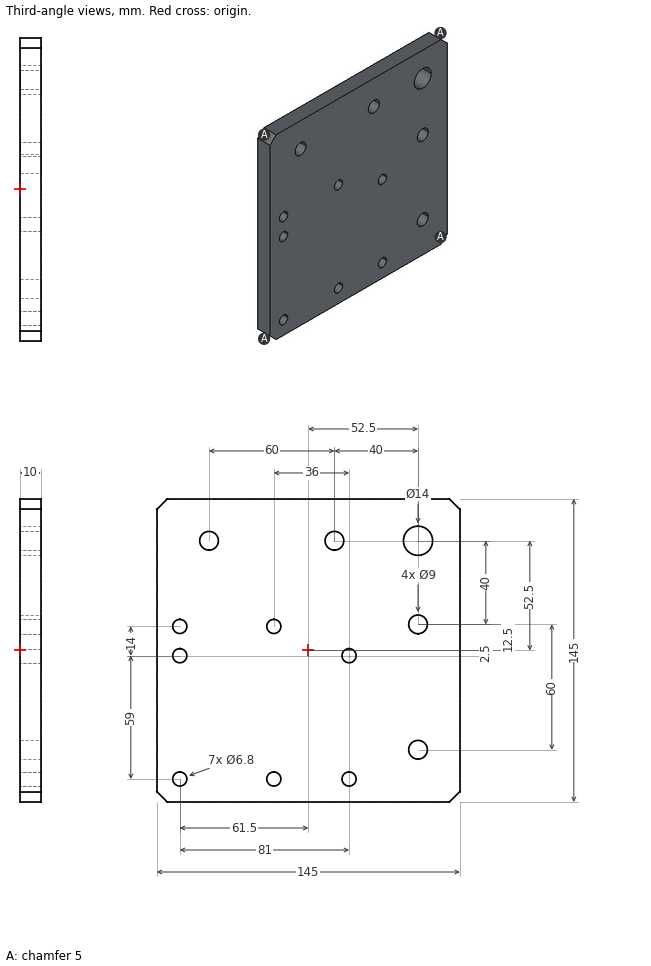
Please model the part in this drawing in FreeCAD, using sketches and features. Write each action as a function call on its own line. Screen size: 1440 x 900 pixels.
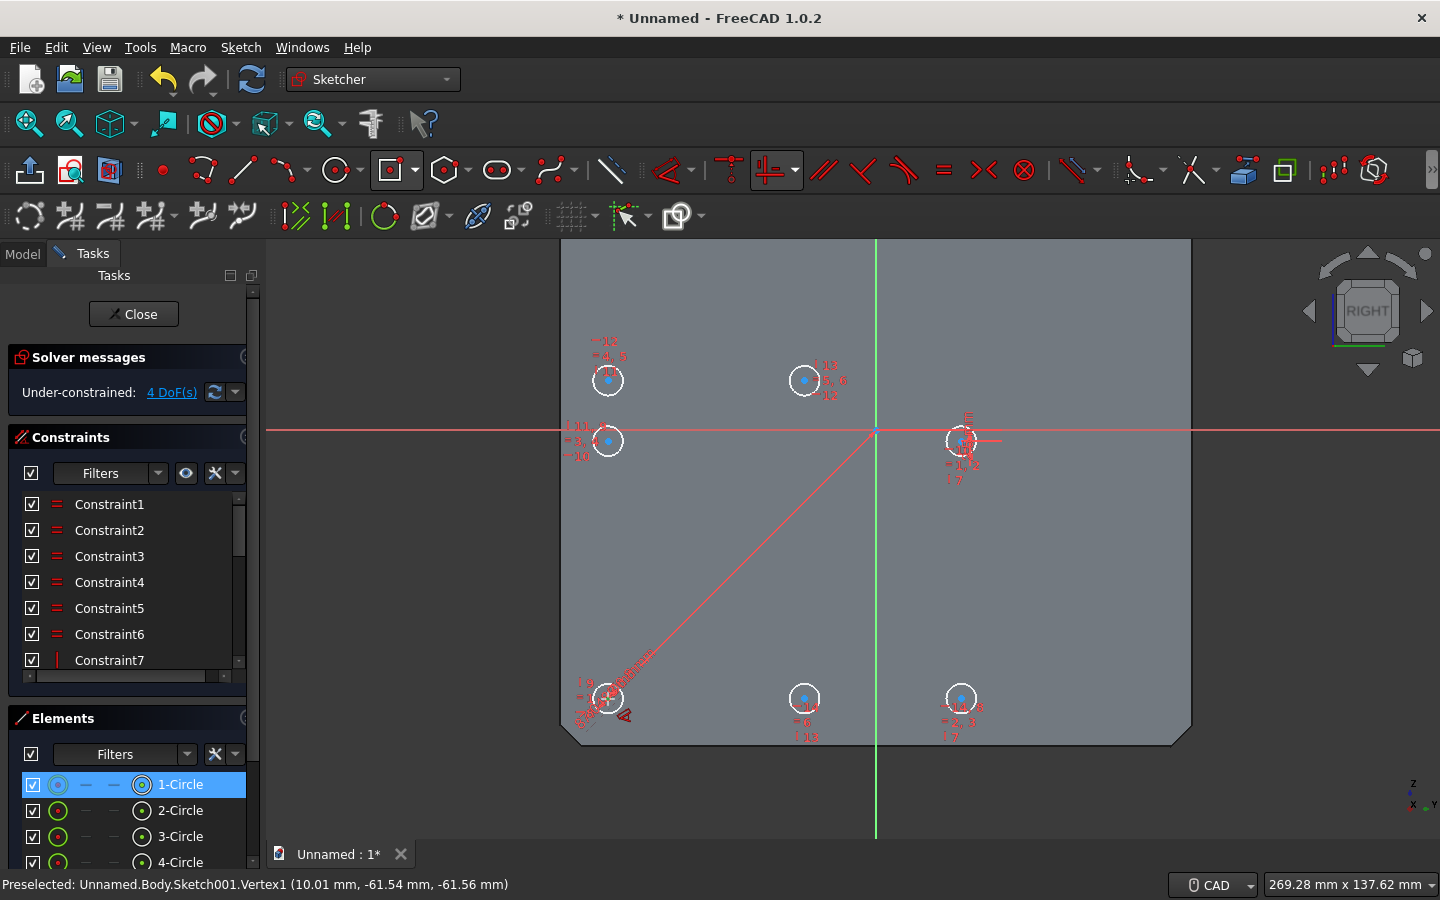
click(961, 441)
click(785, 733)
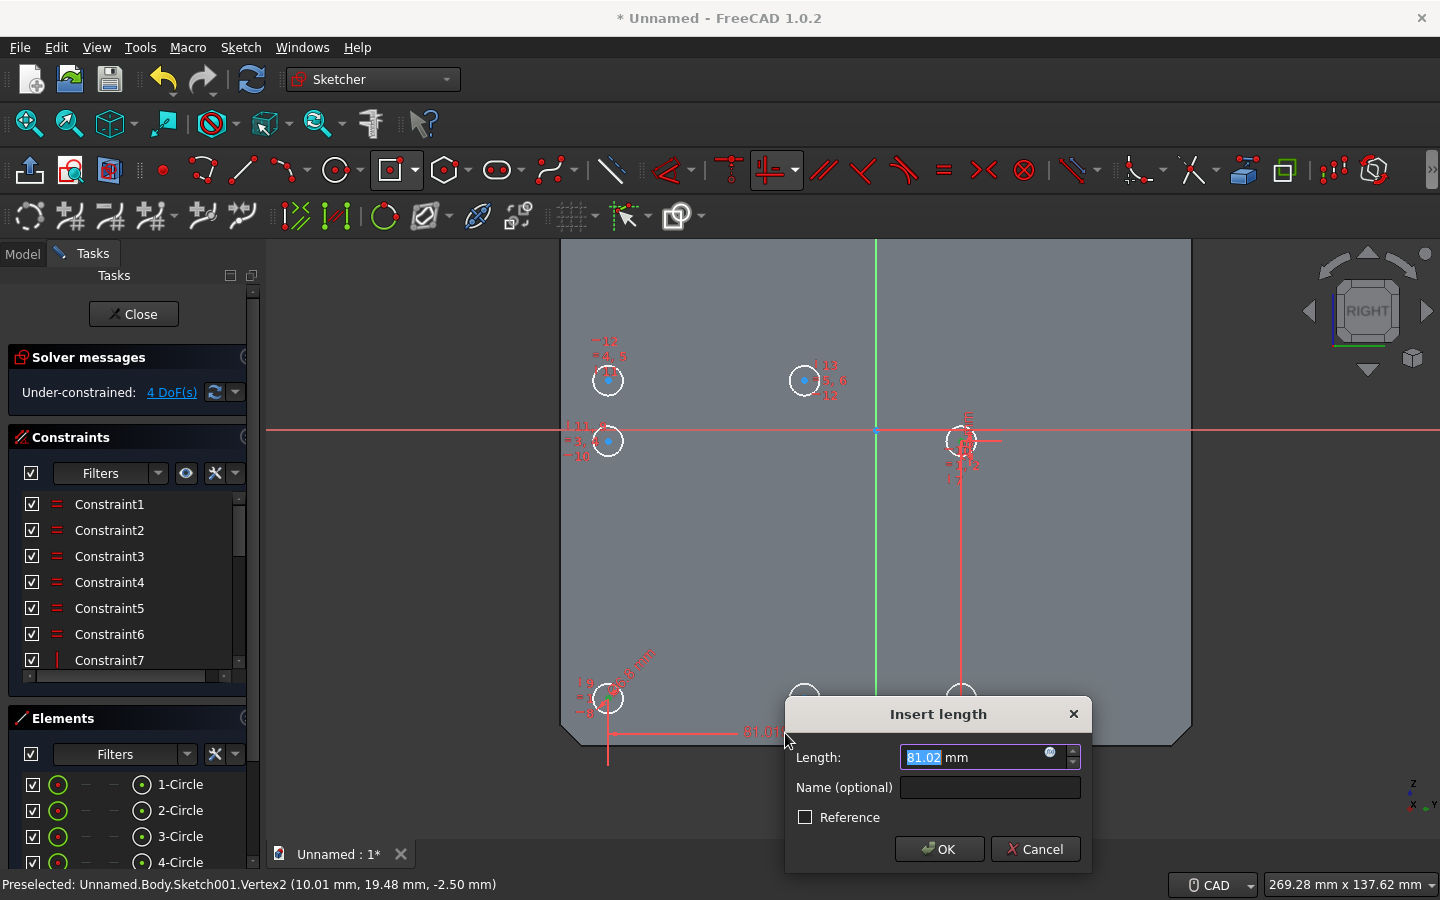
text(81)
key(Return)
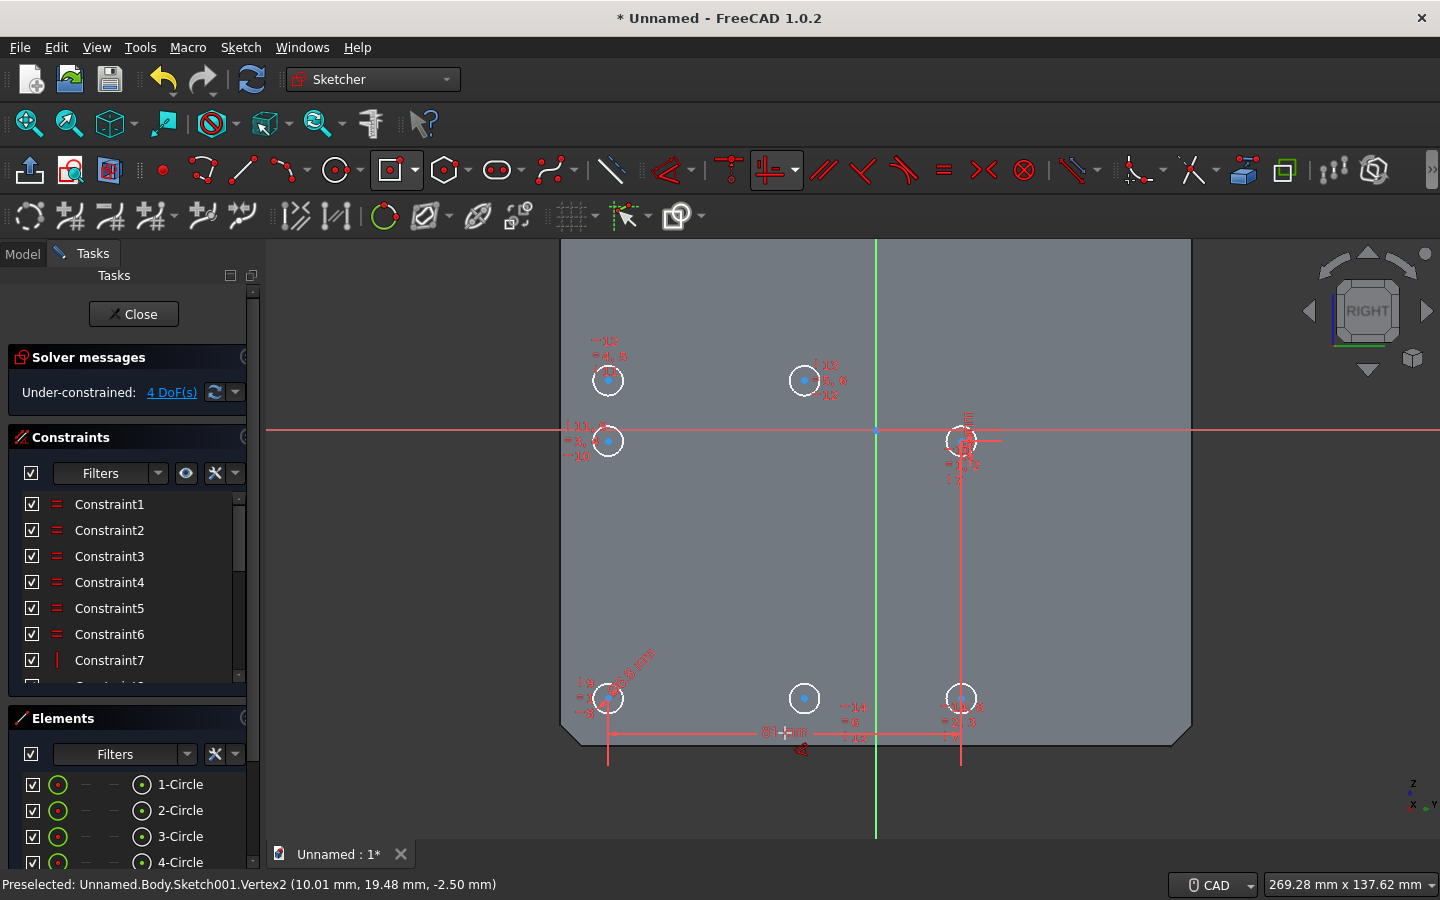
click(608, 699)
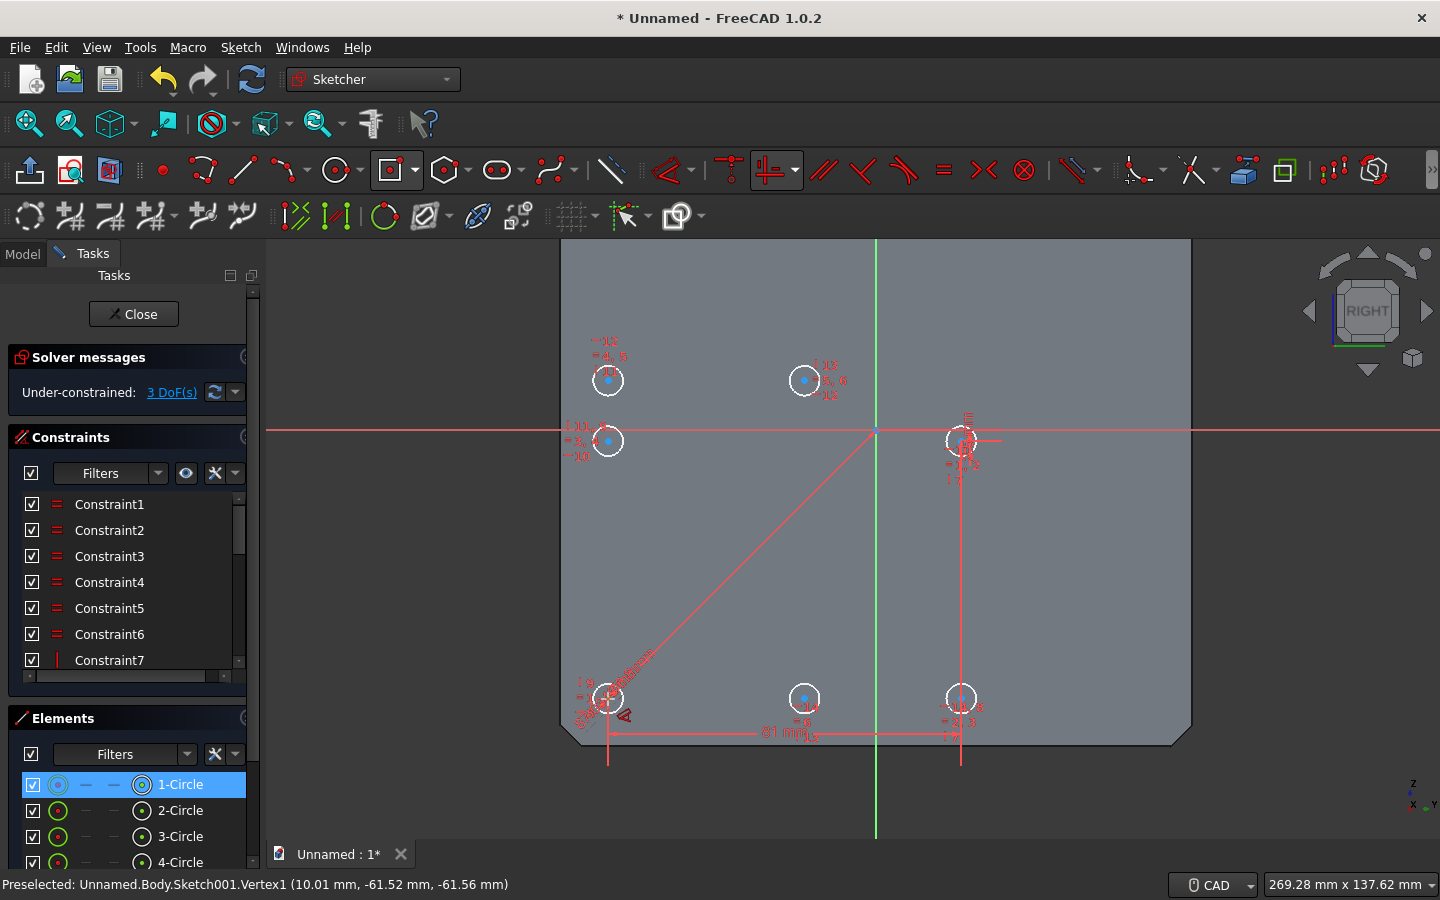
click(961, 441)
click(574, 570)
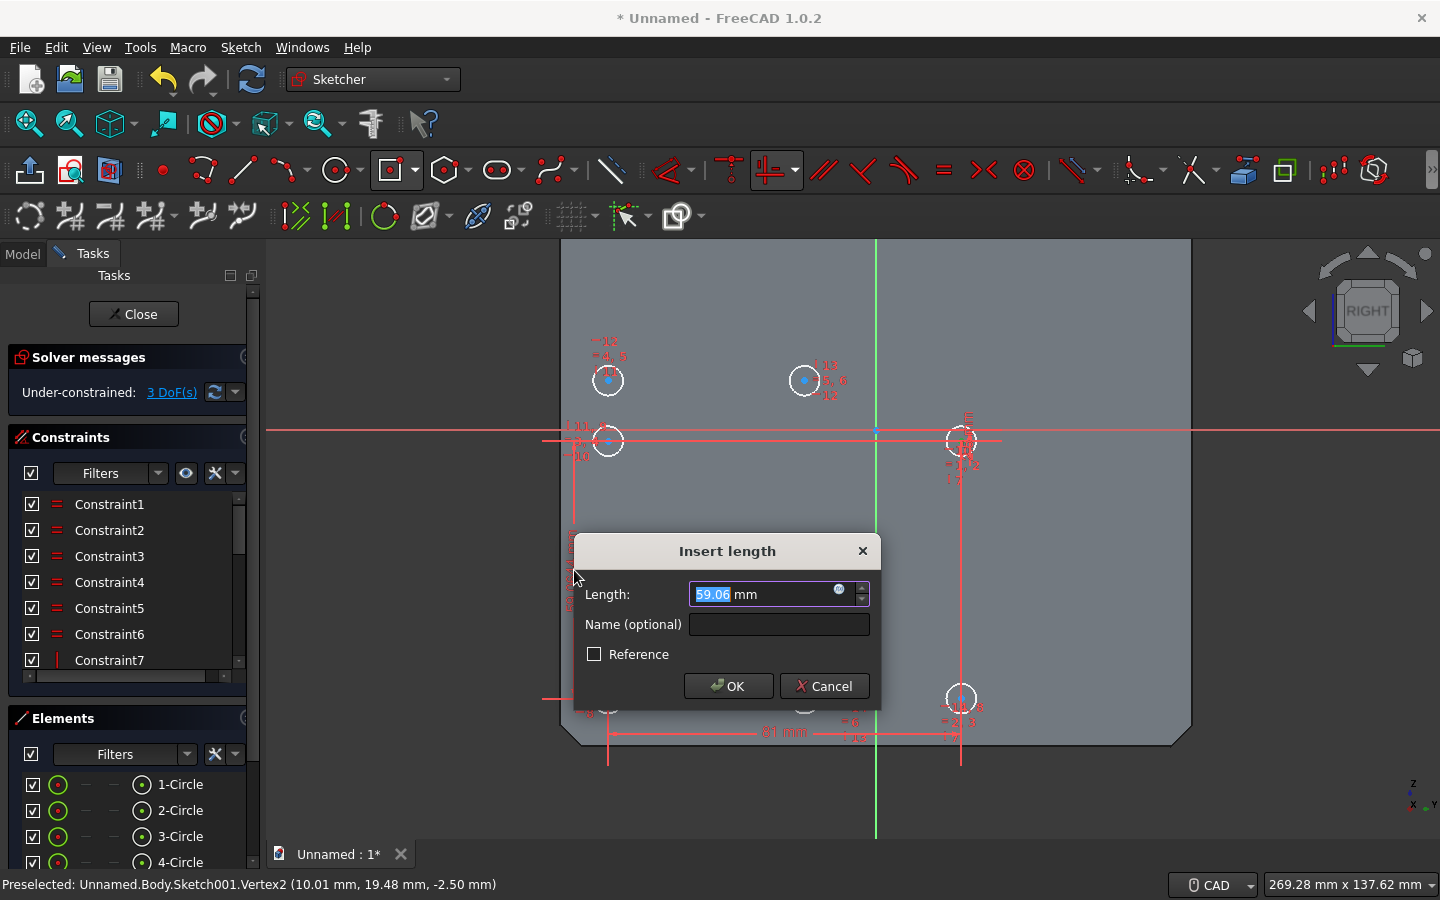
text(59)
key(Return)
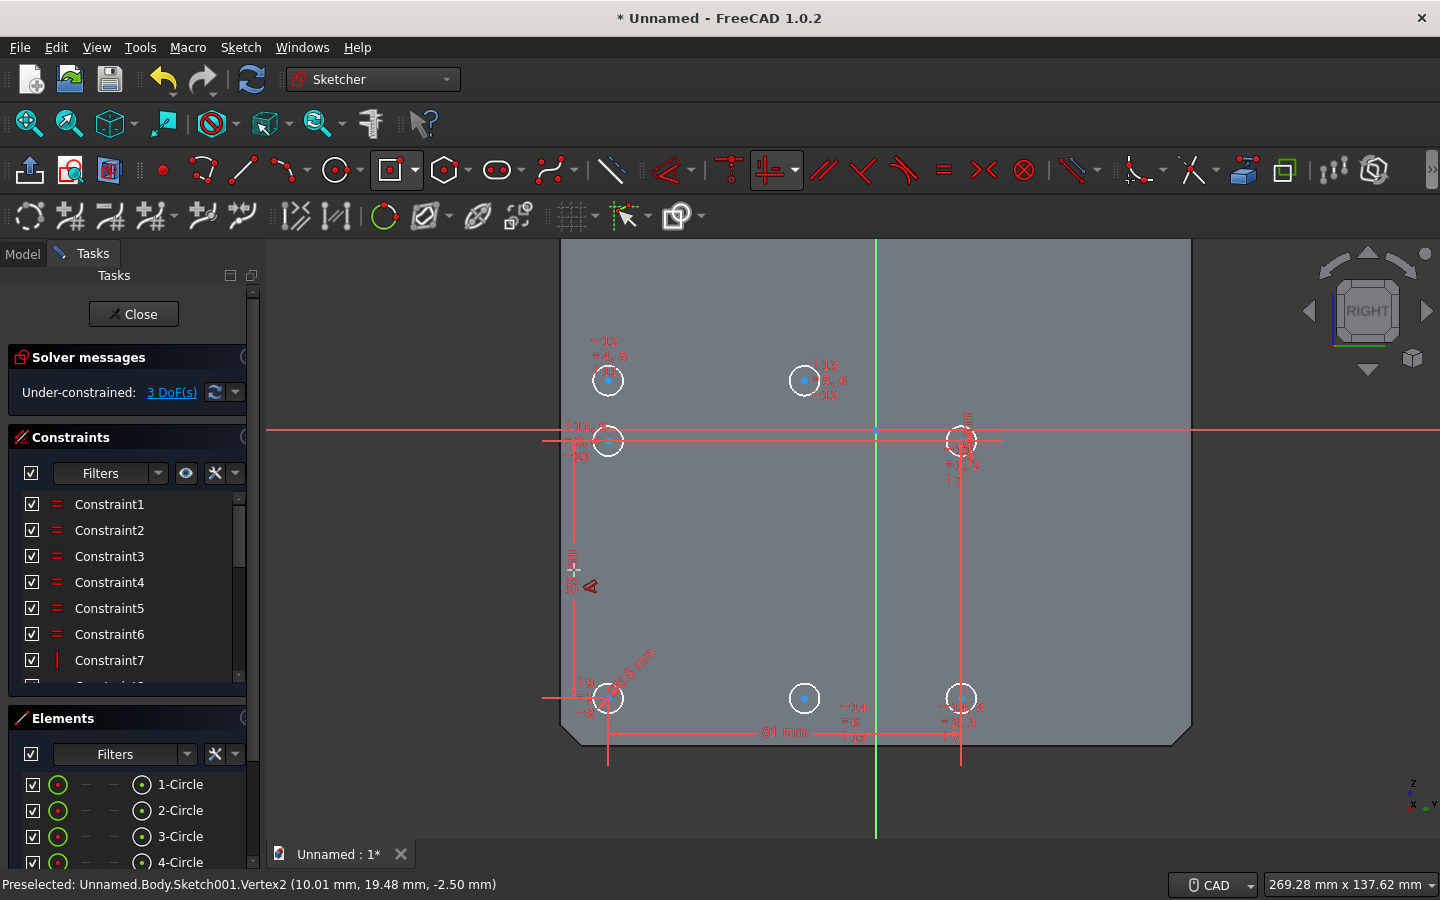
click(608, 441)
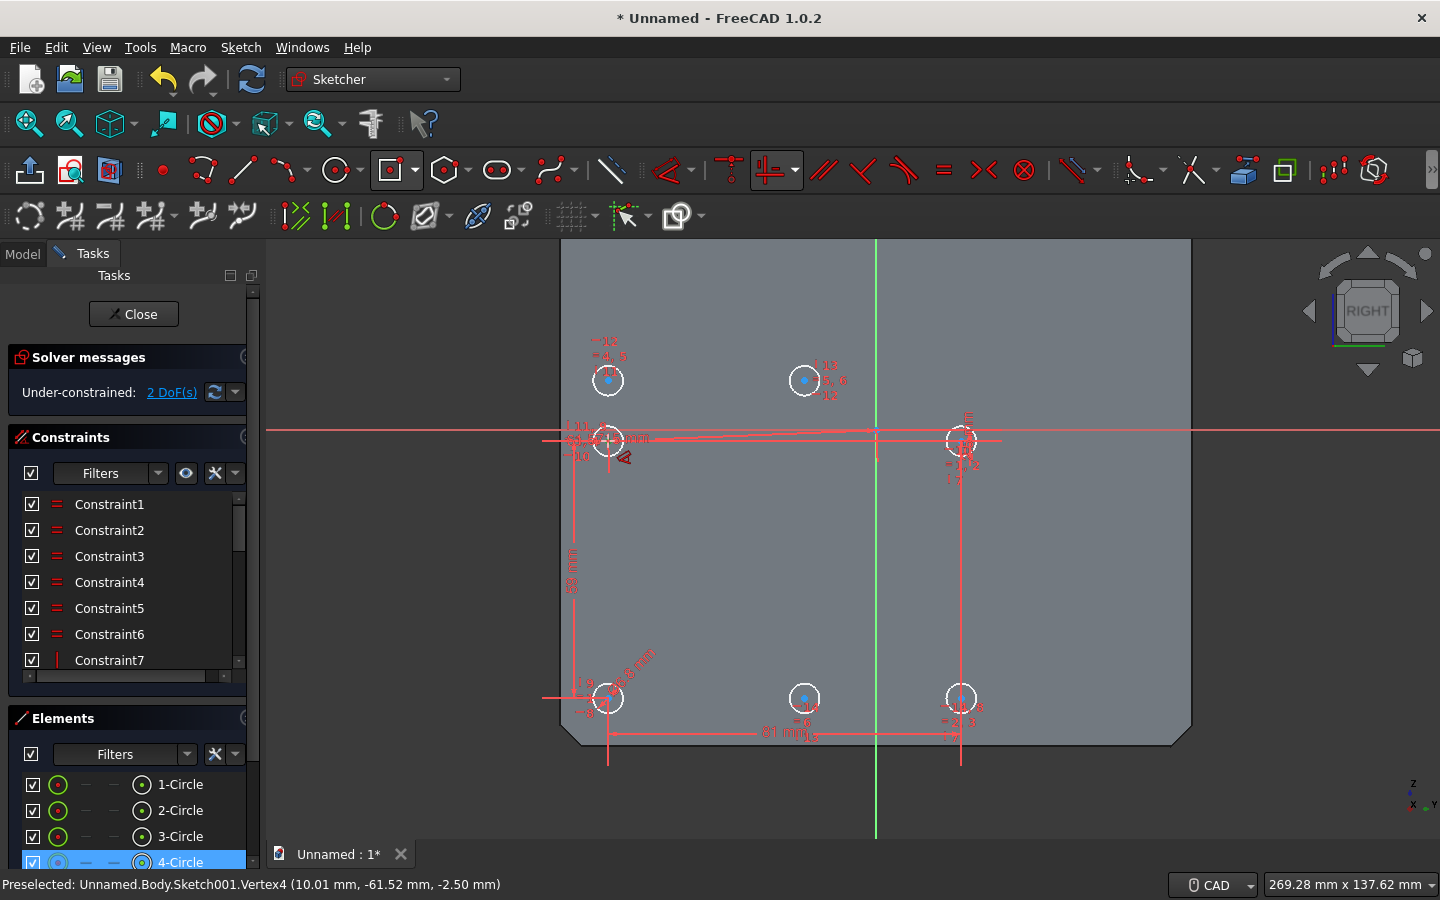
click(608, 381)
click(574, 411)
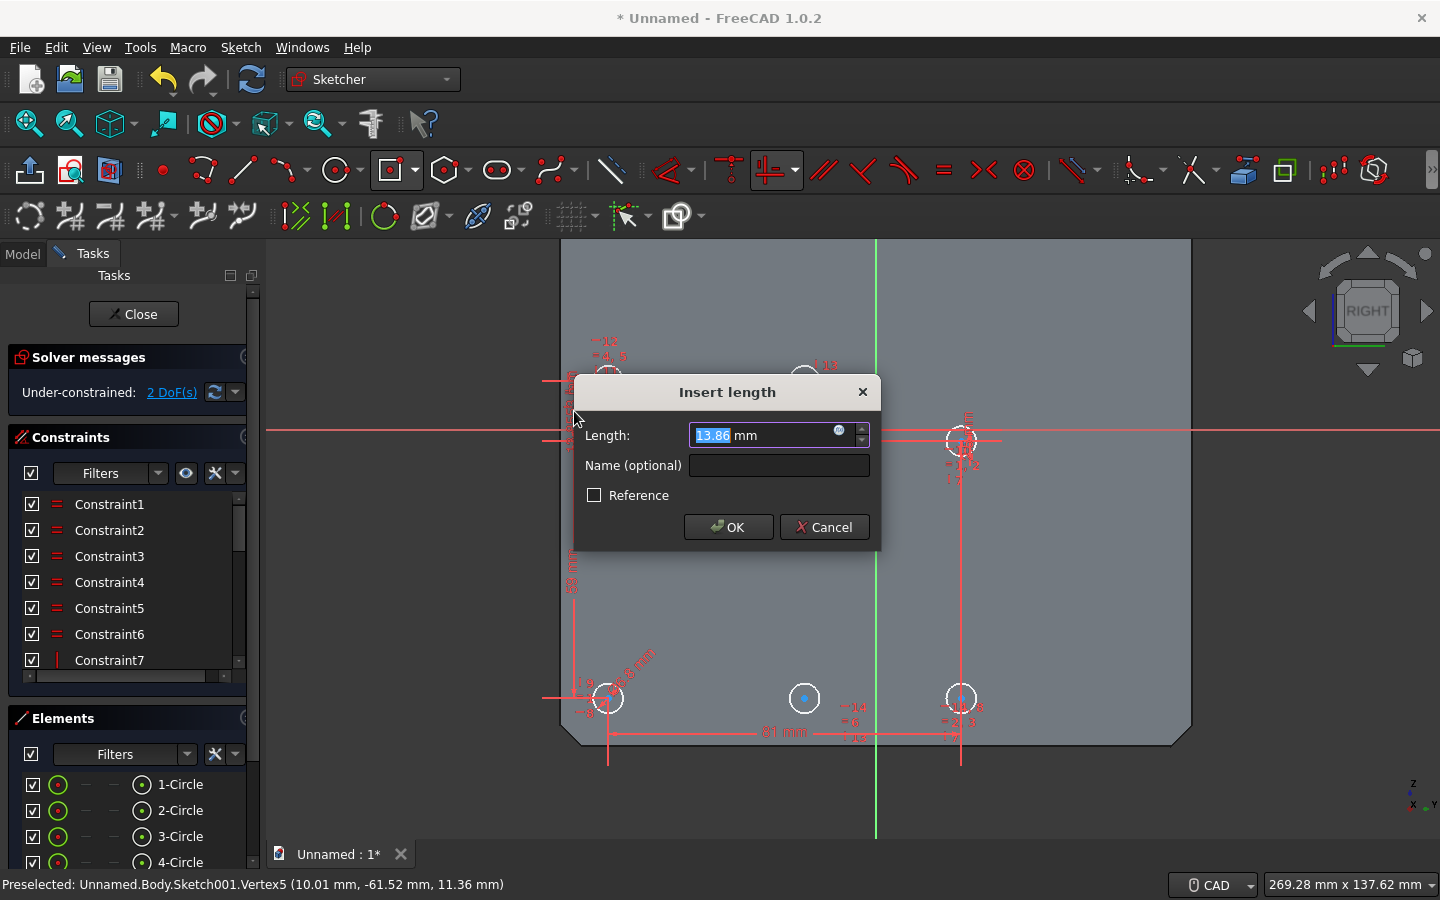
text(14)
key(Return)